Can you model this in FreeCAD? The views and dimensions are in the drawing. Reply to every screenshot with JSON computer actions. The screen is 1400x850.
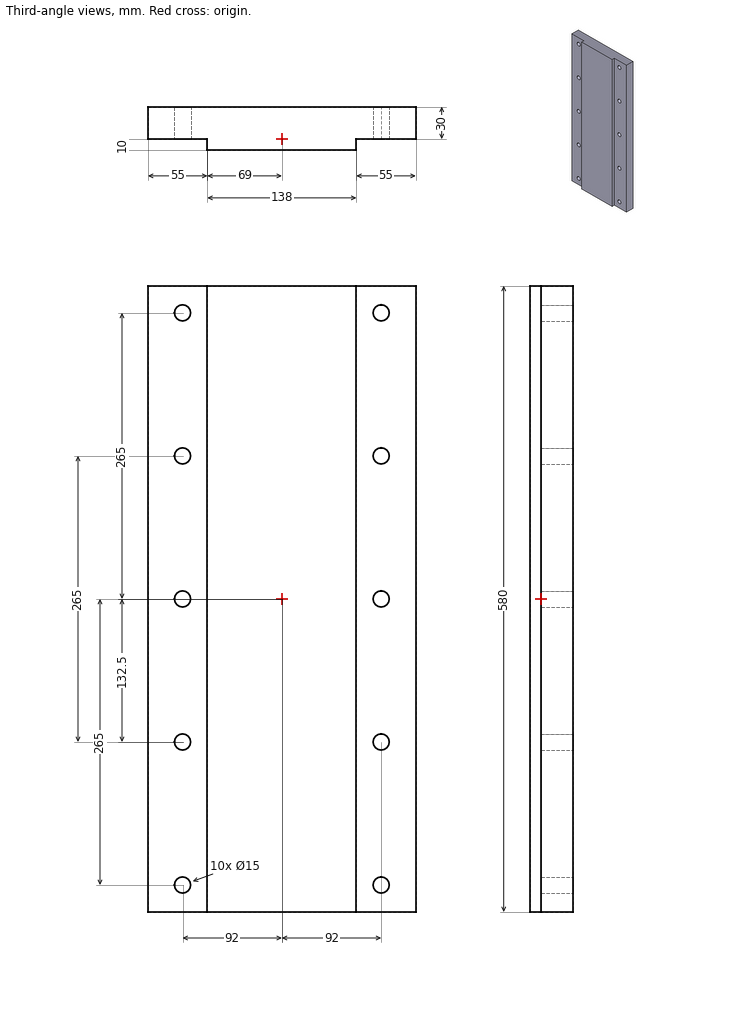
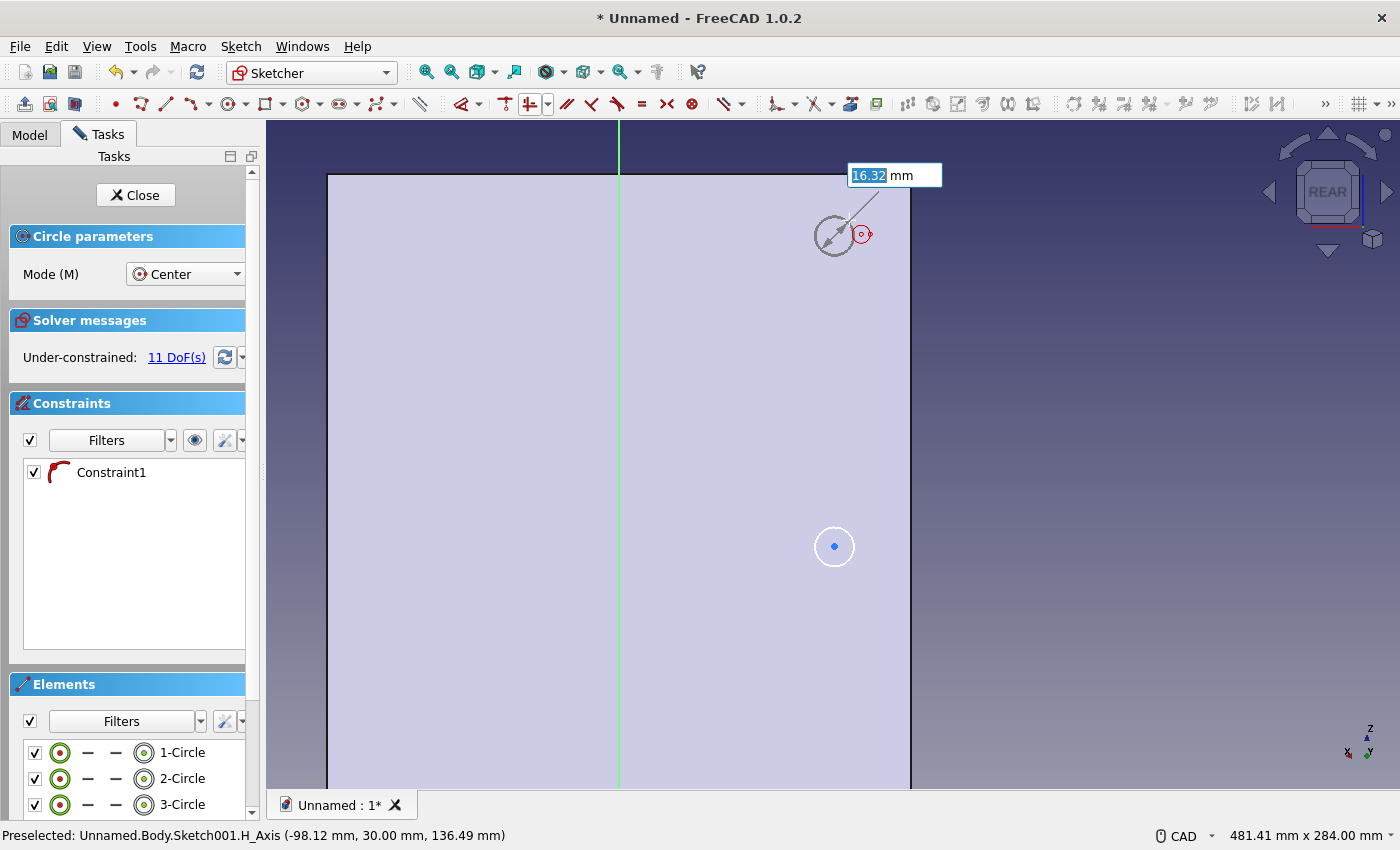
{"action": "left_click", "coordinate": [848, 220]}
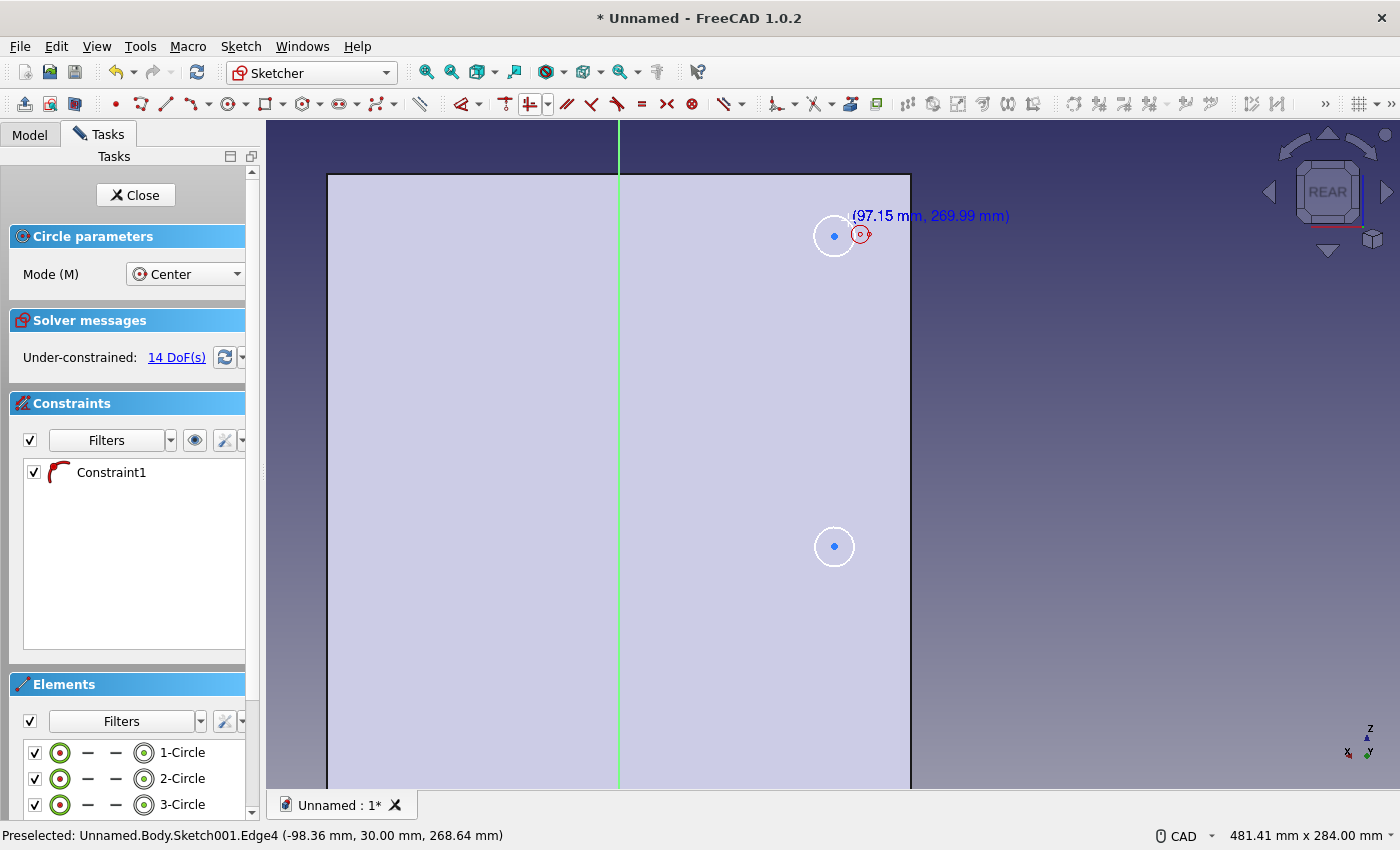
{"action": "scroll", "coordinate": [849, 220], "scroll_direction": "down", "scroll_amount": 5}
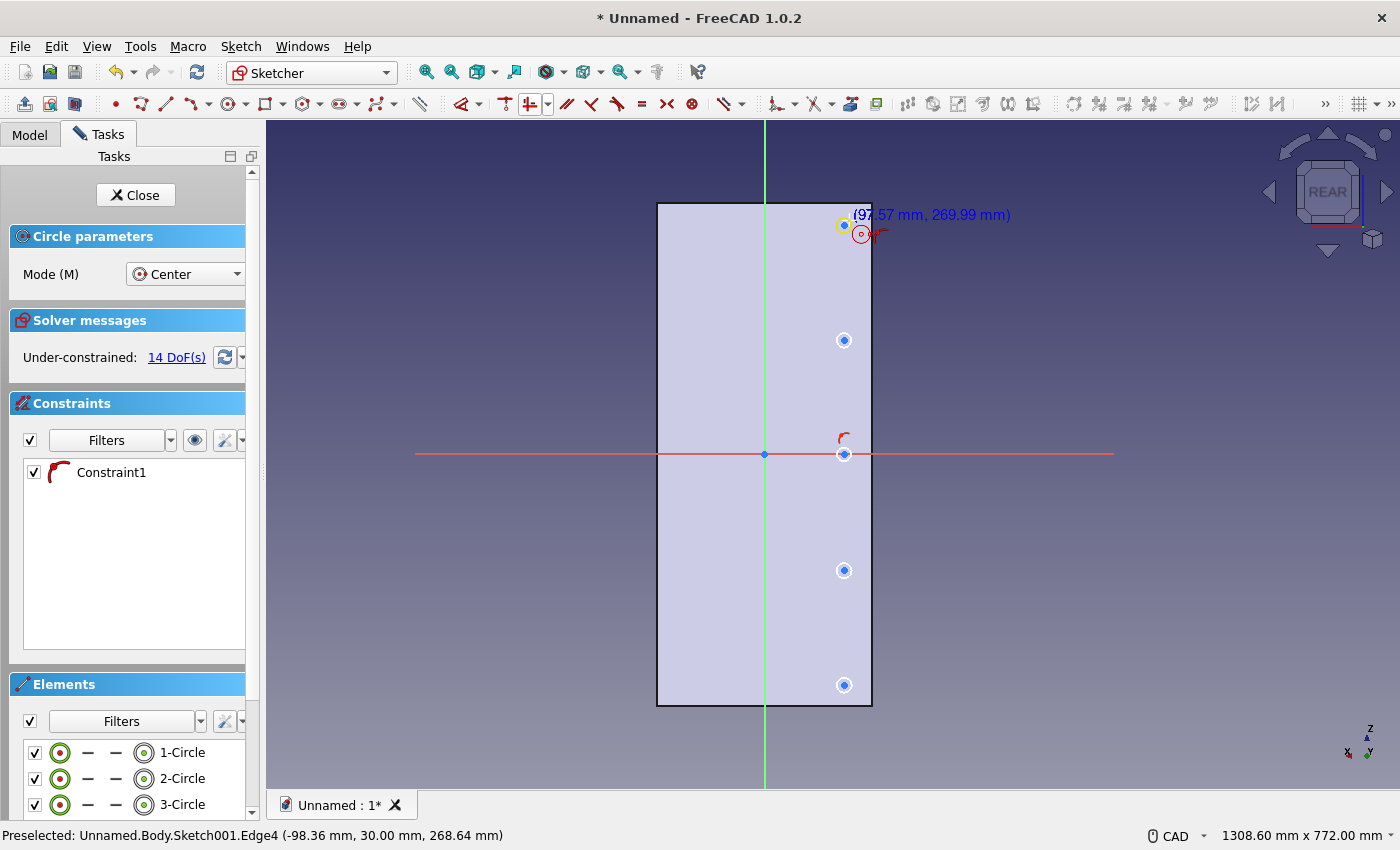
{"action": "scroll", "coordinate": [685, 569], "scroll_direction": "up", "scroll_amount": 7}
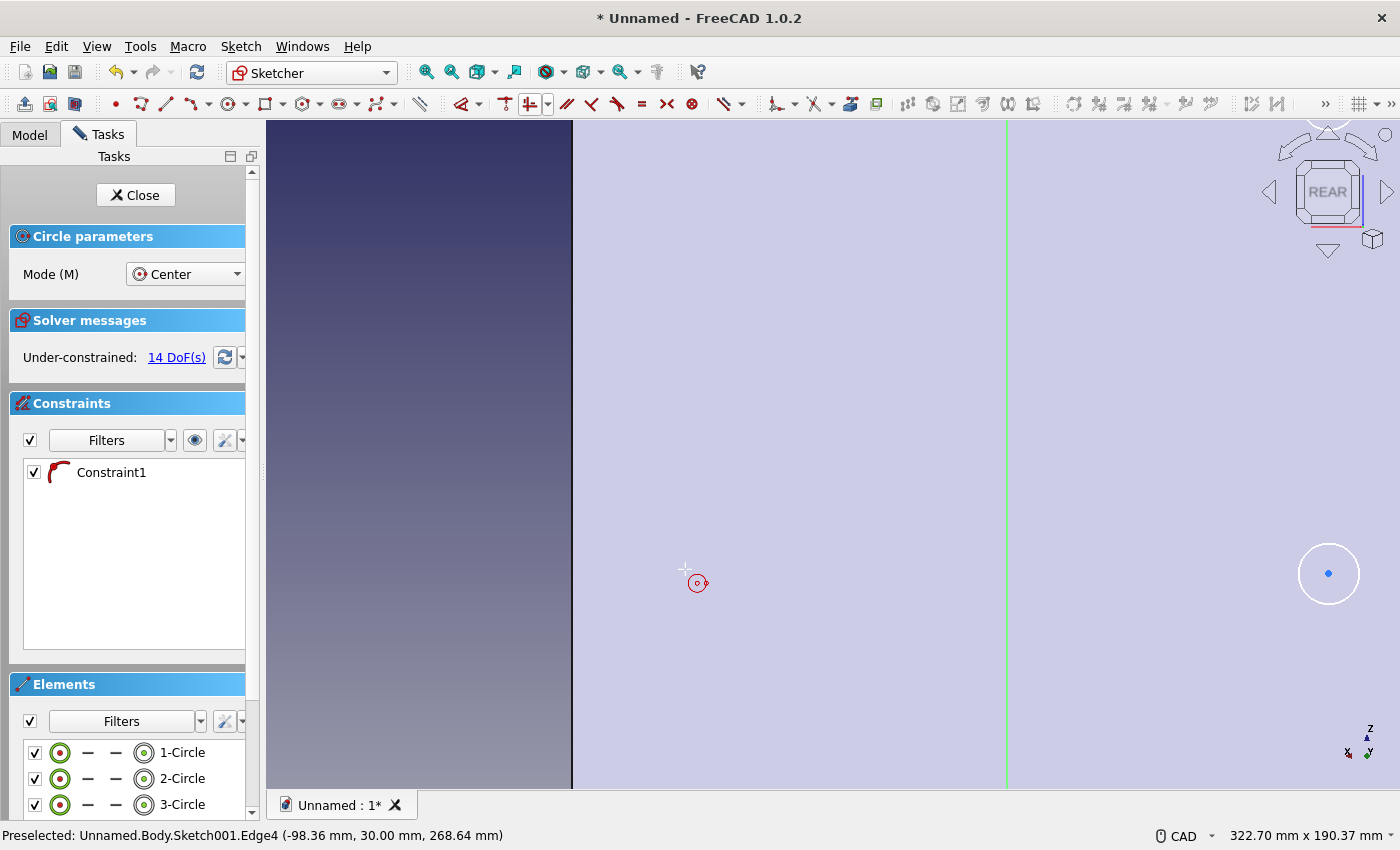
{"action": "scroll", "coordinate": [685, 570], "scroll_direction": "down", "scroll_amount": 7}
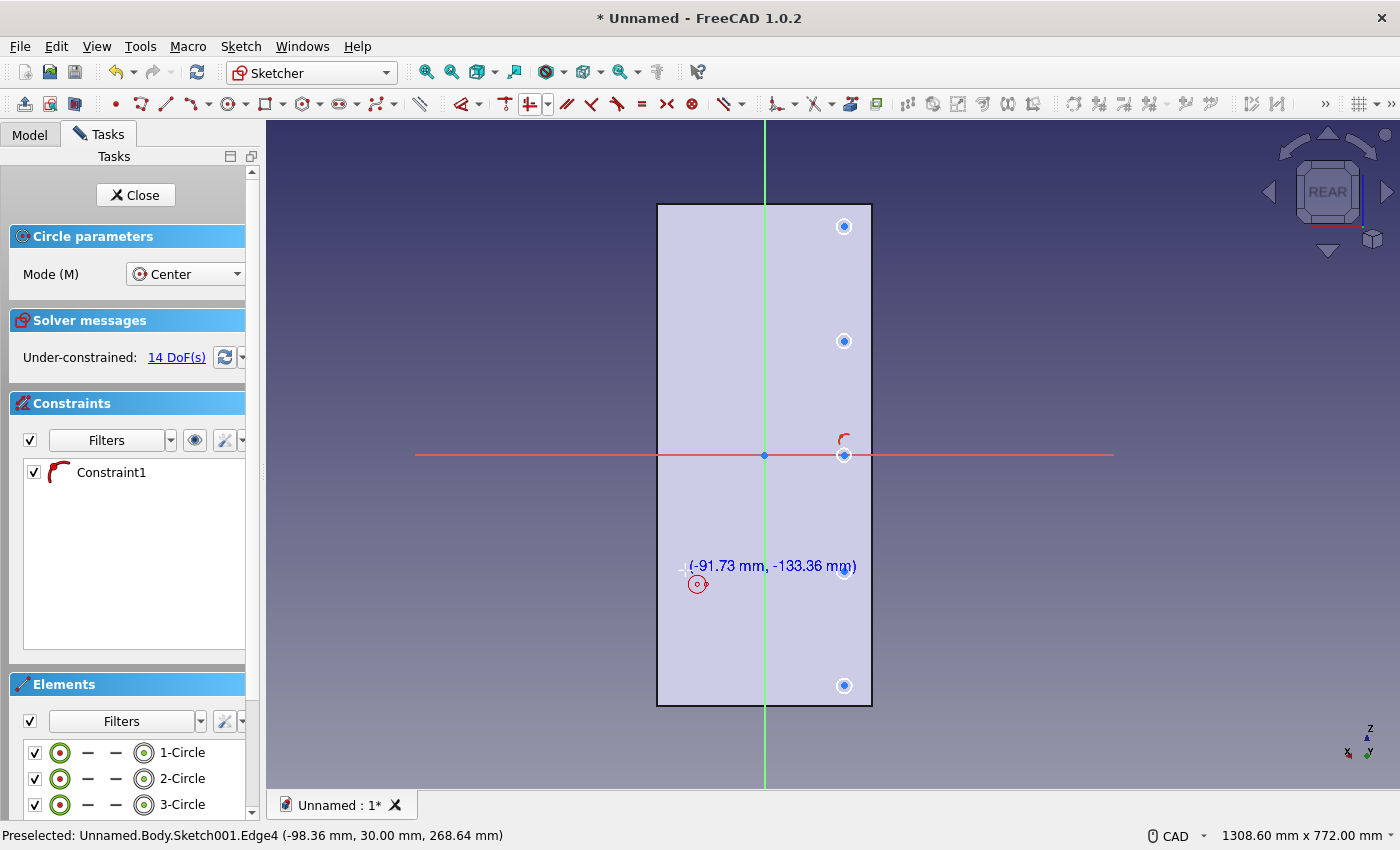
{"action": "left_click", "coordinate": [685, 570]}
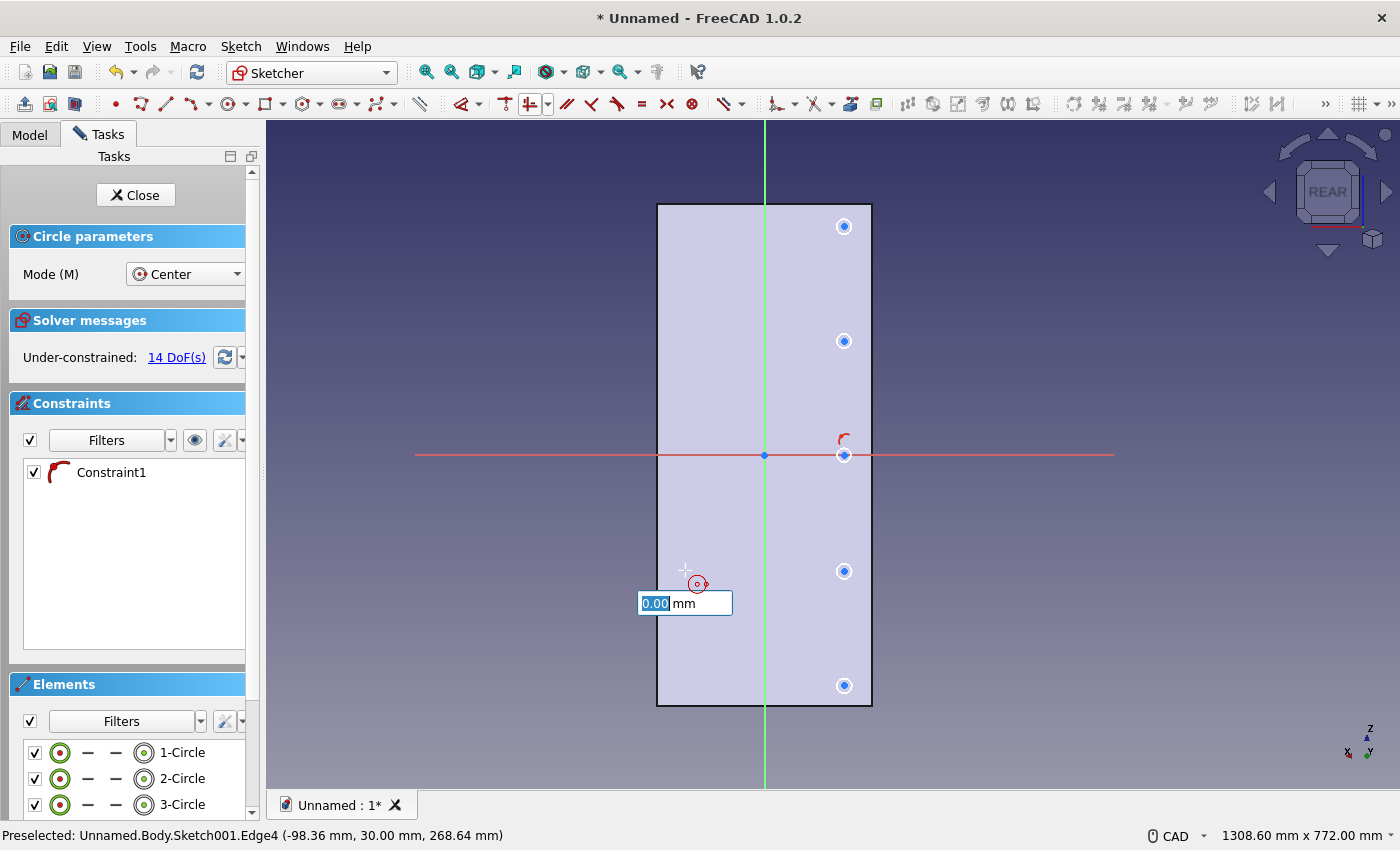
{"action": "scroll", "coordinate": [690, 565], "scroll_direction": "up", "scroll_amount": 5}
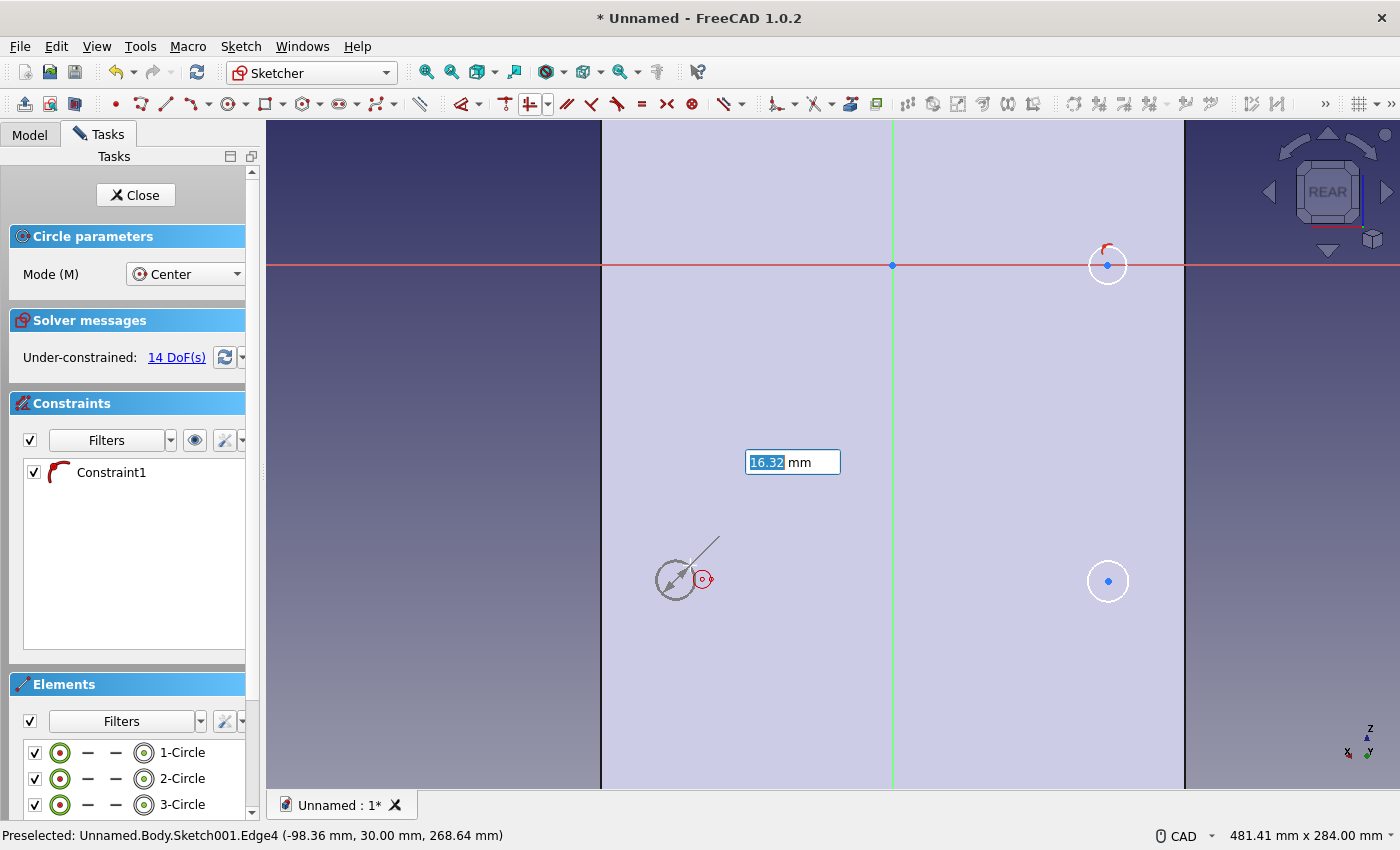
{"action": "left_click", "coordinate": [688, 565]}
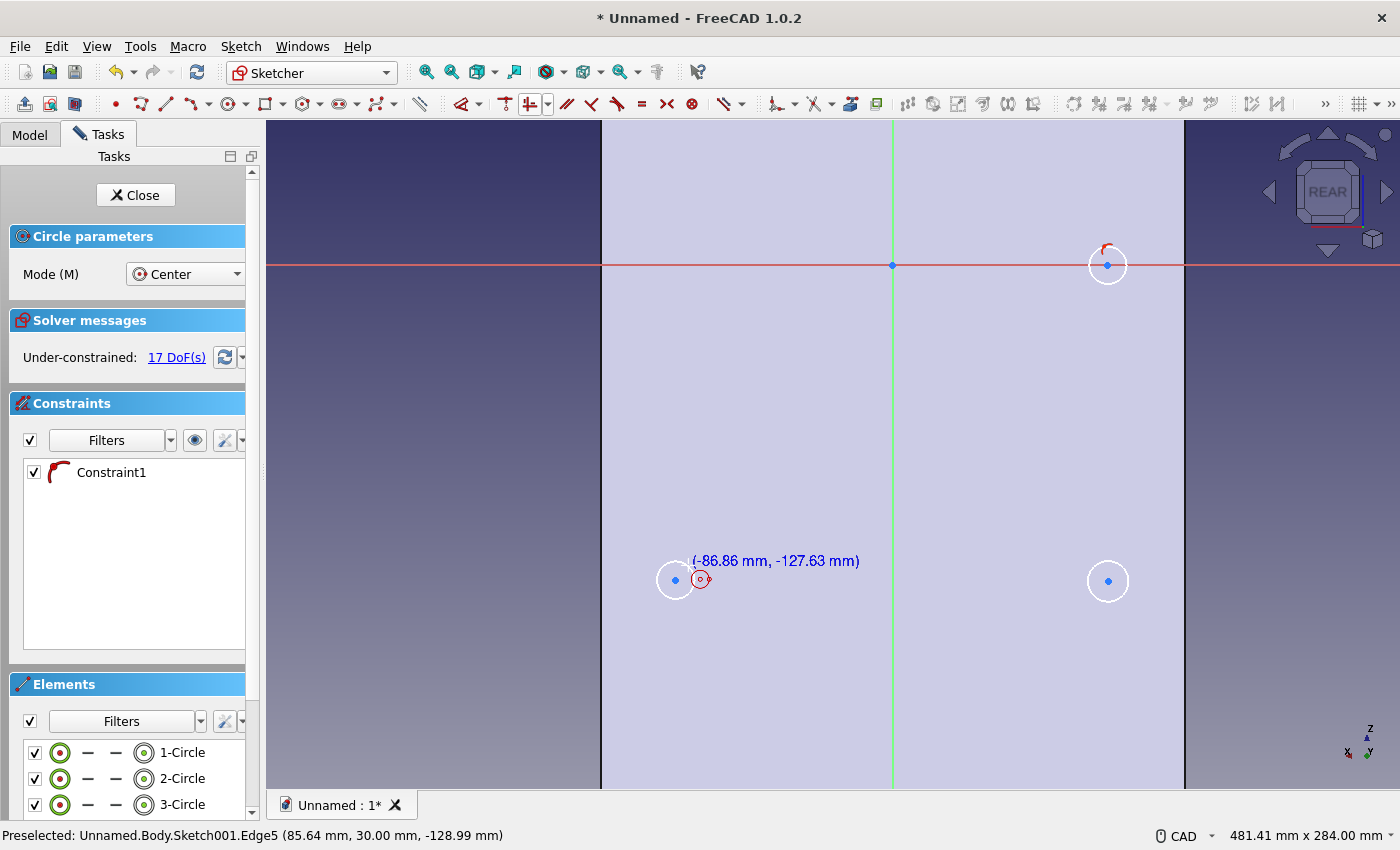
{"action": "scroll", "coordinate": [676, 265], "scroll_direction": "up", "scroll_amount": 2}